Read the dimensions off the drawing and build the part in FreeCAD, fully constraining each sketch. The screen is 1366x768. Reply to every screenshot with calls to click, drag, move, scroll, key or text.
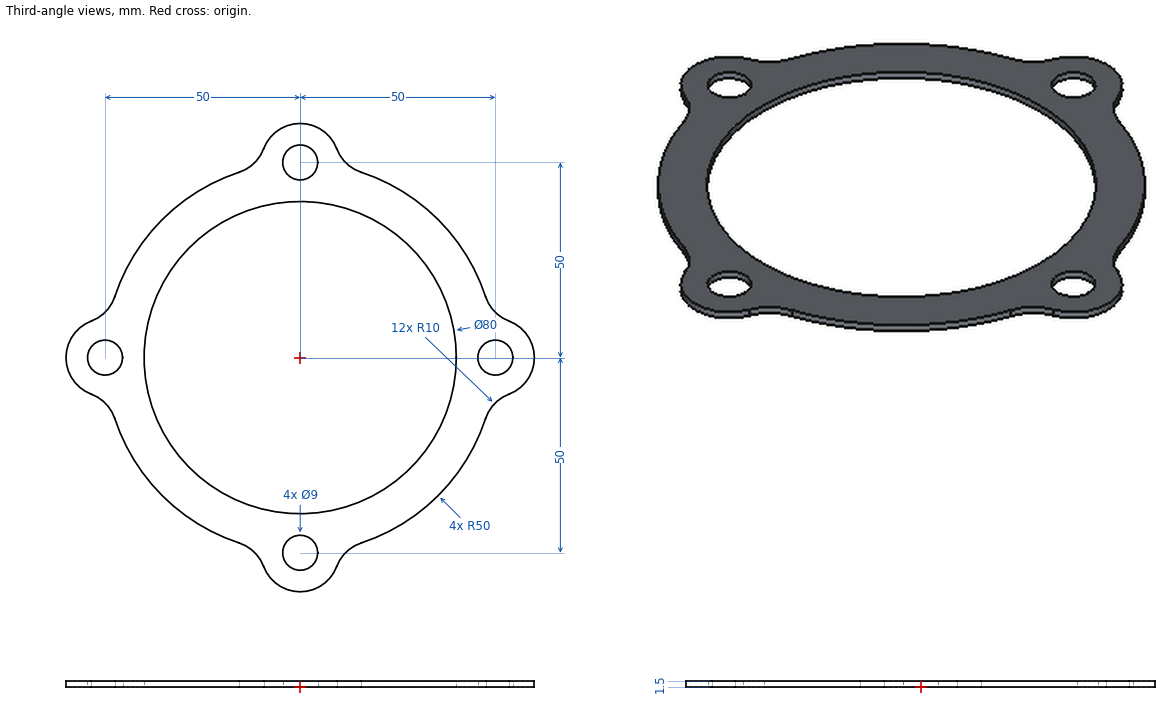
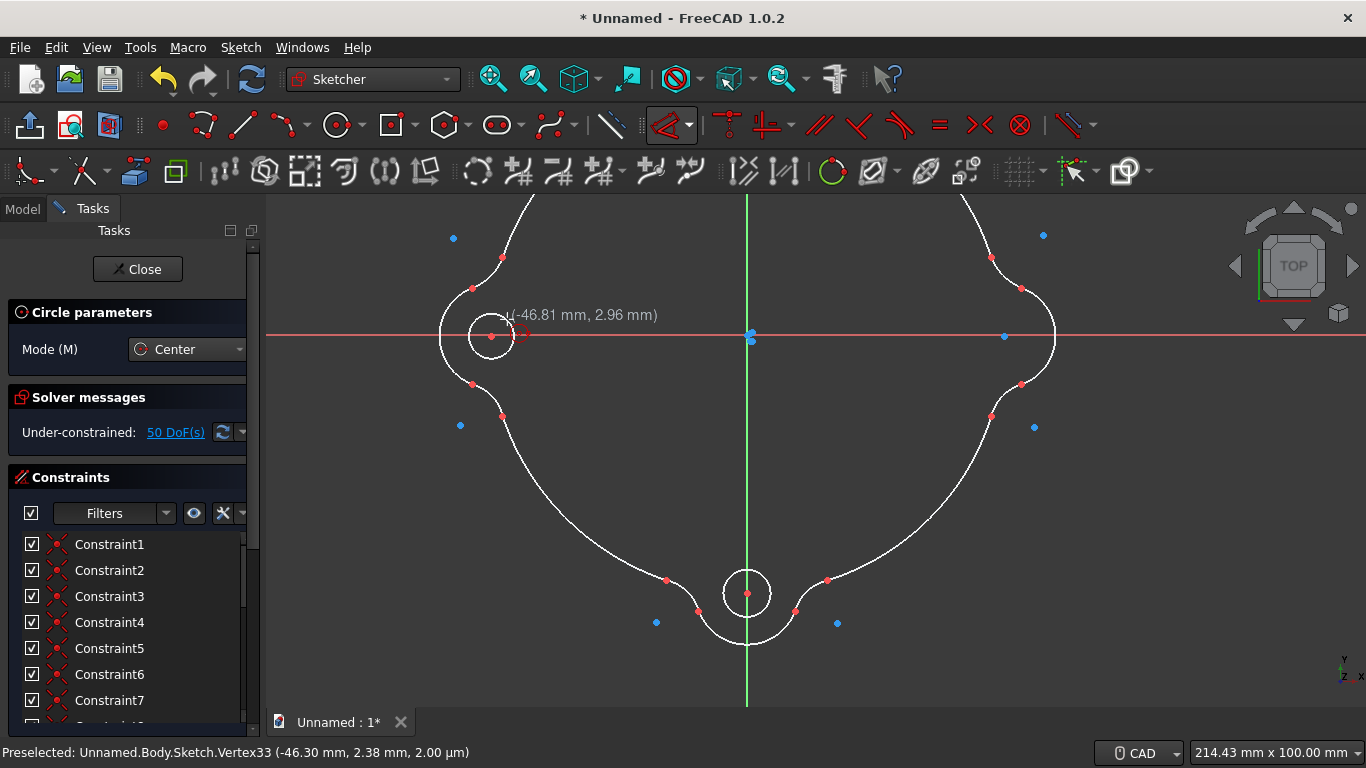
click(747, 335)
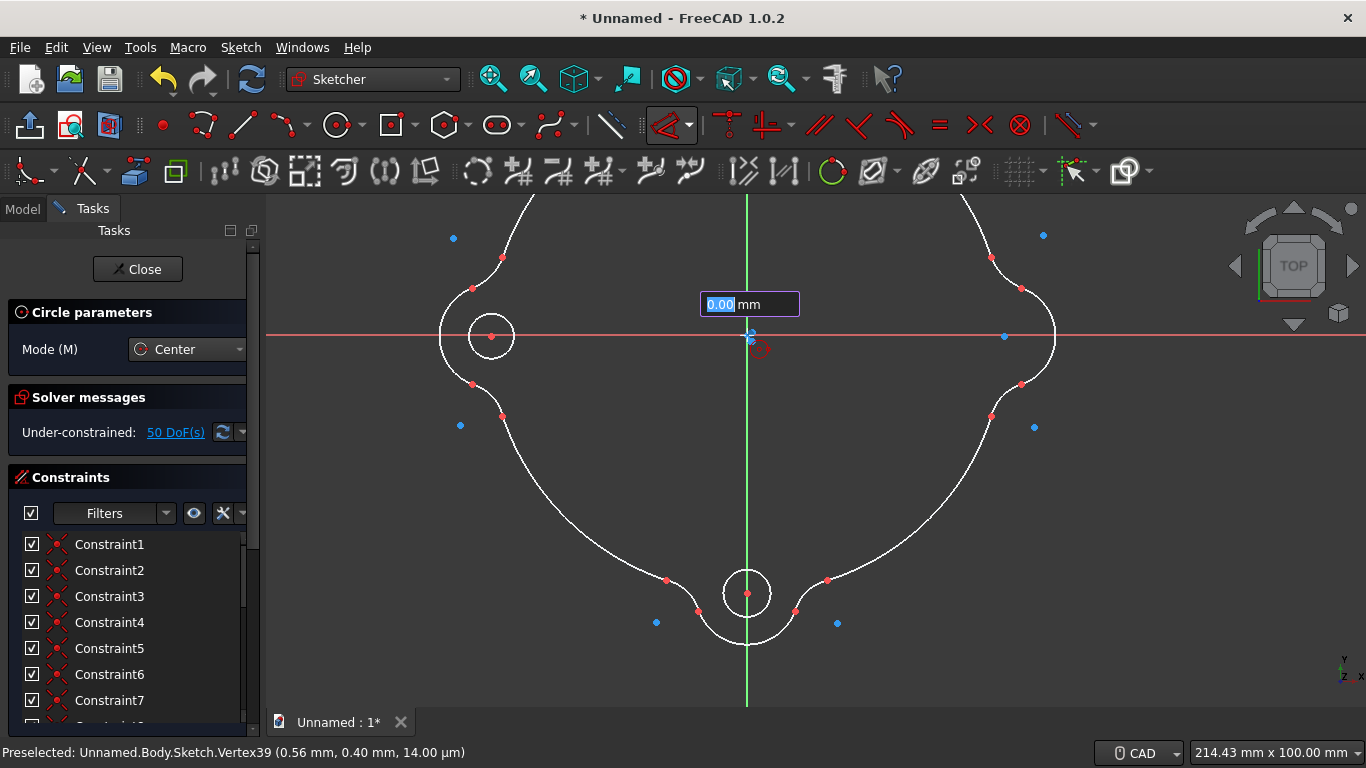
scroll(748, 591, down, 3)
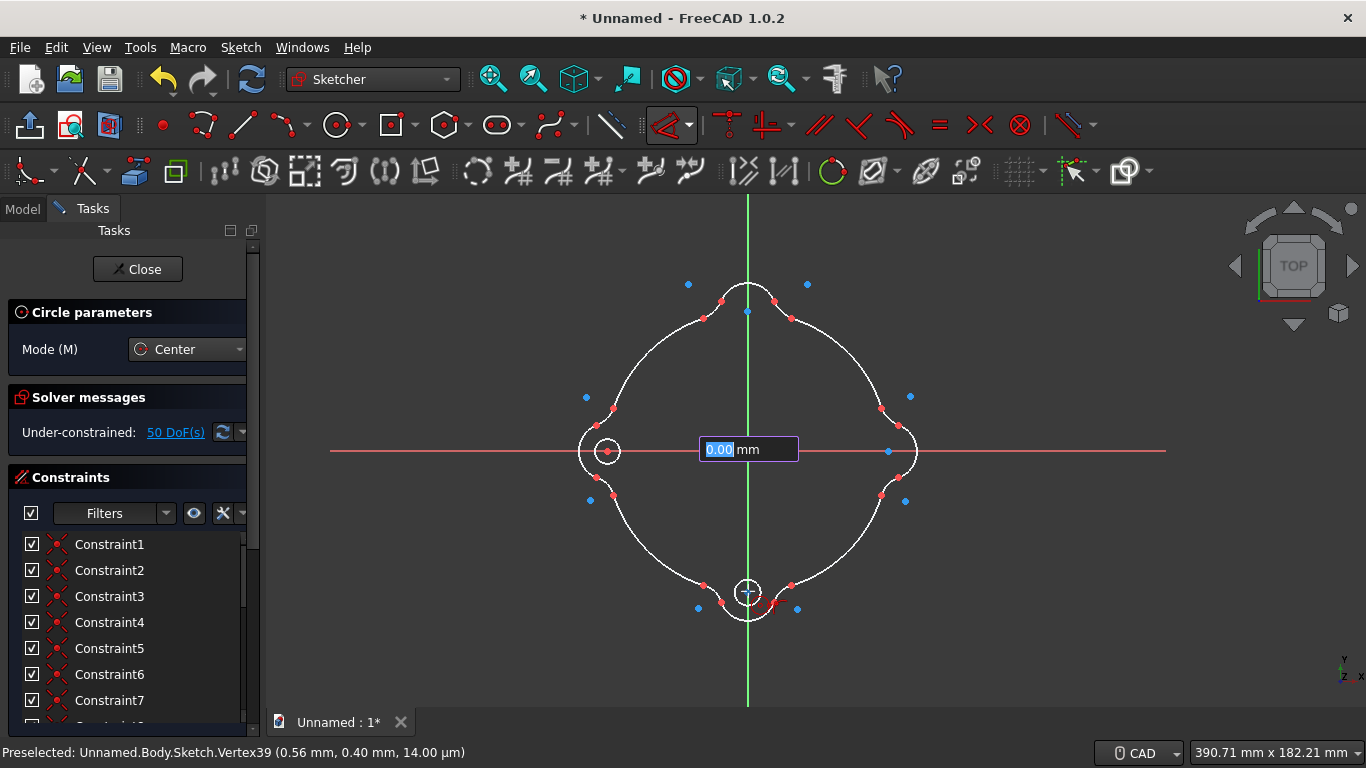
click(827, 371)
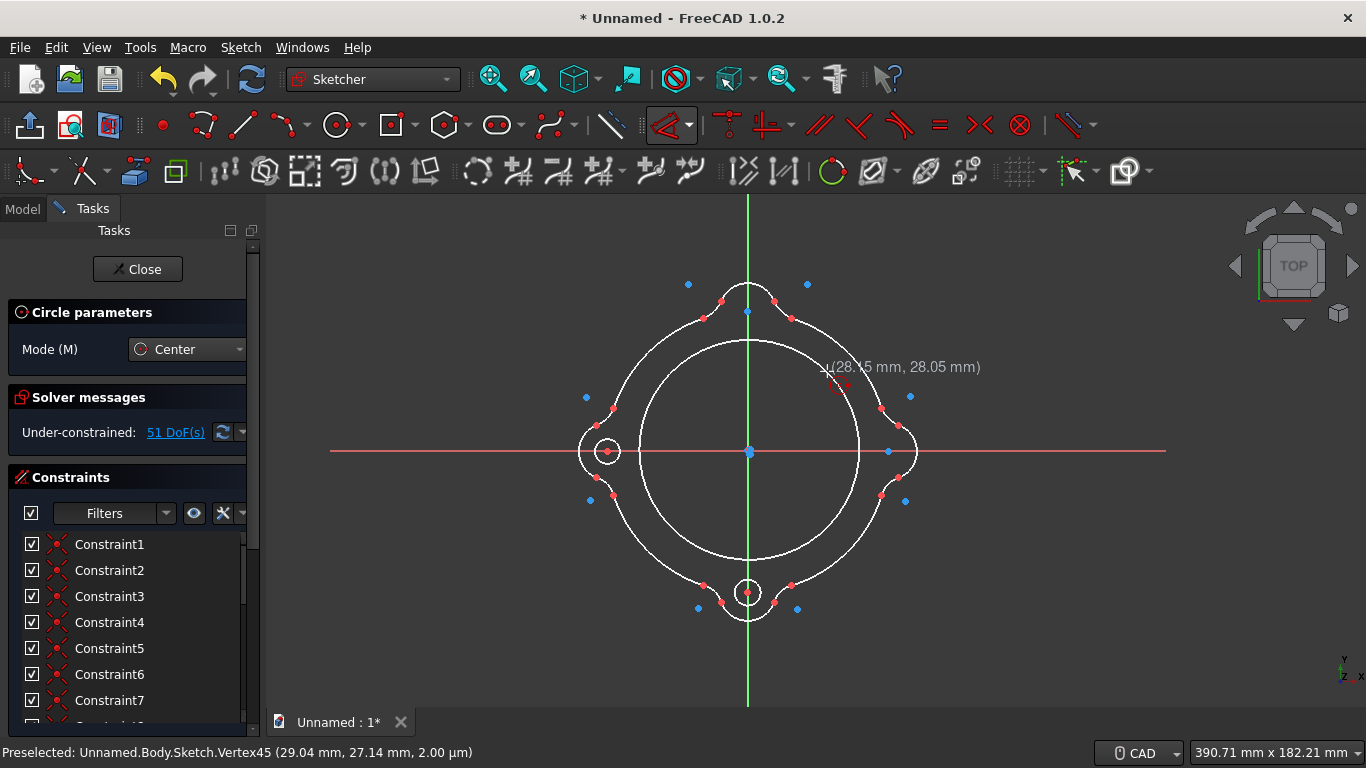
scroll(889, 451, up, 3)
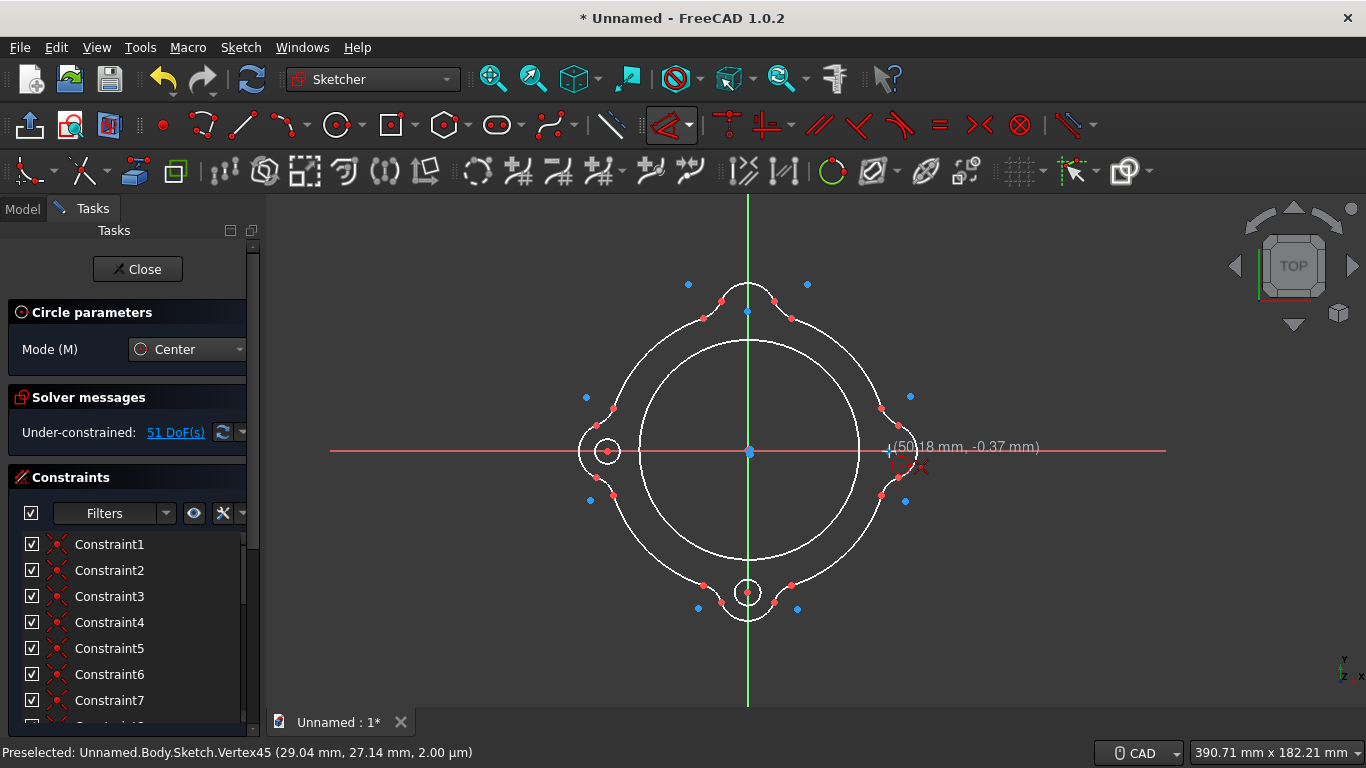
click(888, 451)
click(904, 434)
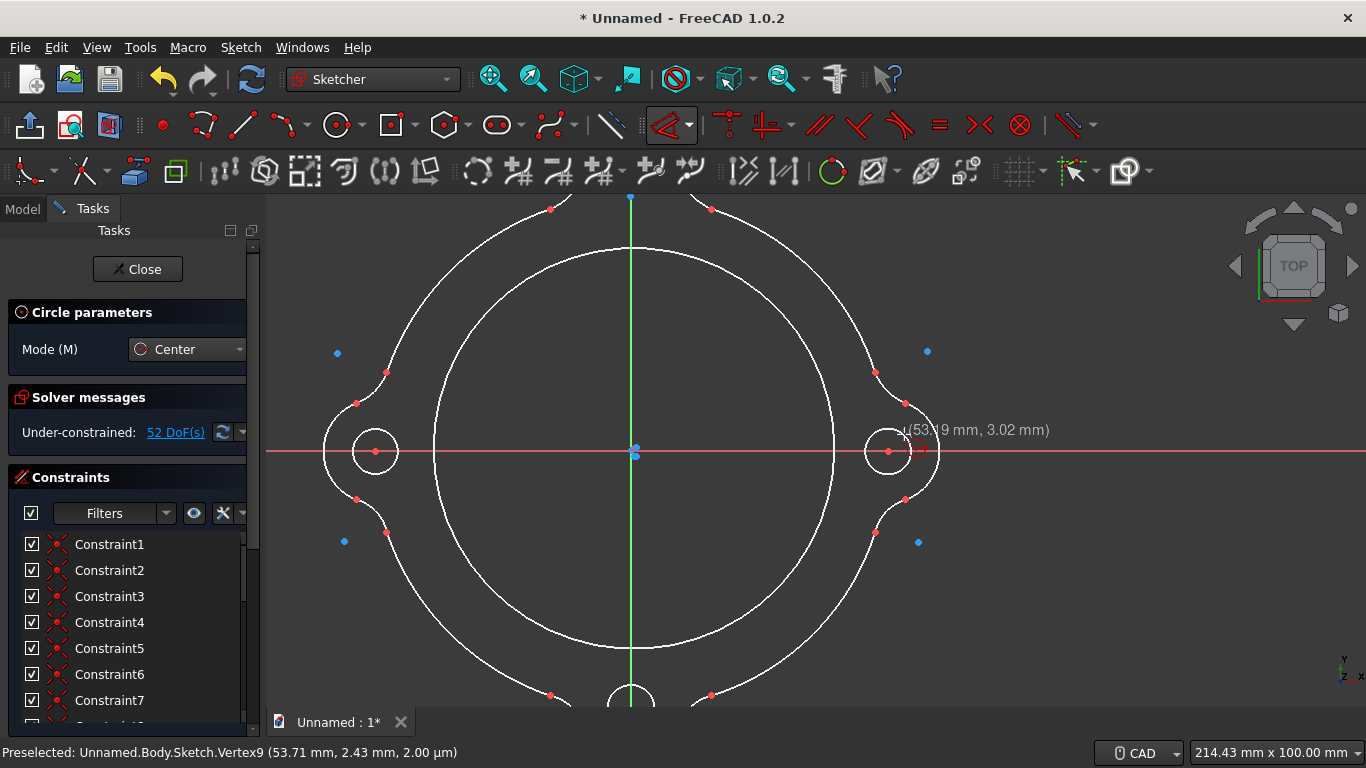
scroll(889, 450, down, 3)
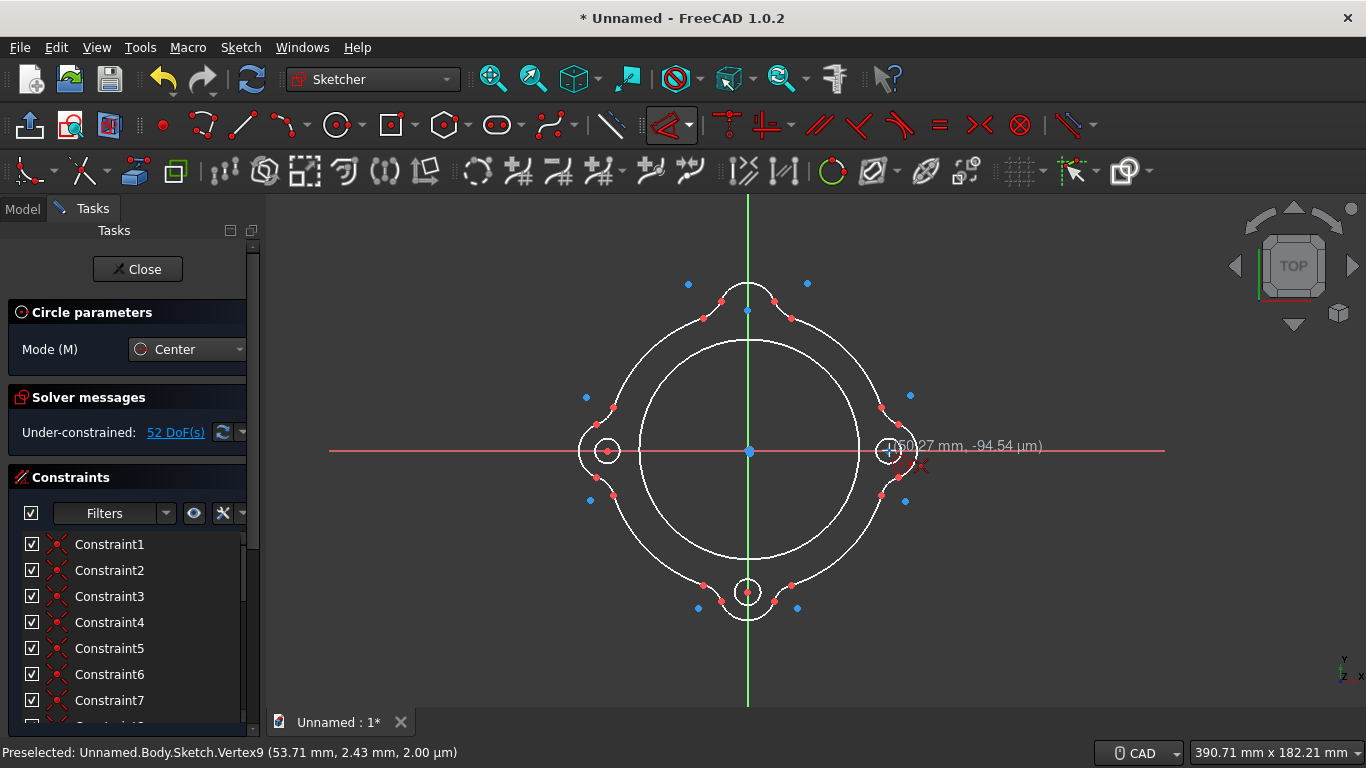
scroll(748, 310, up, 3)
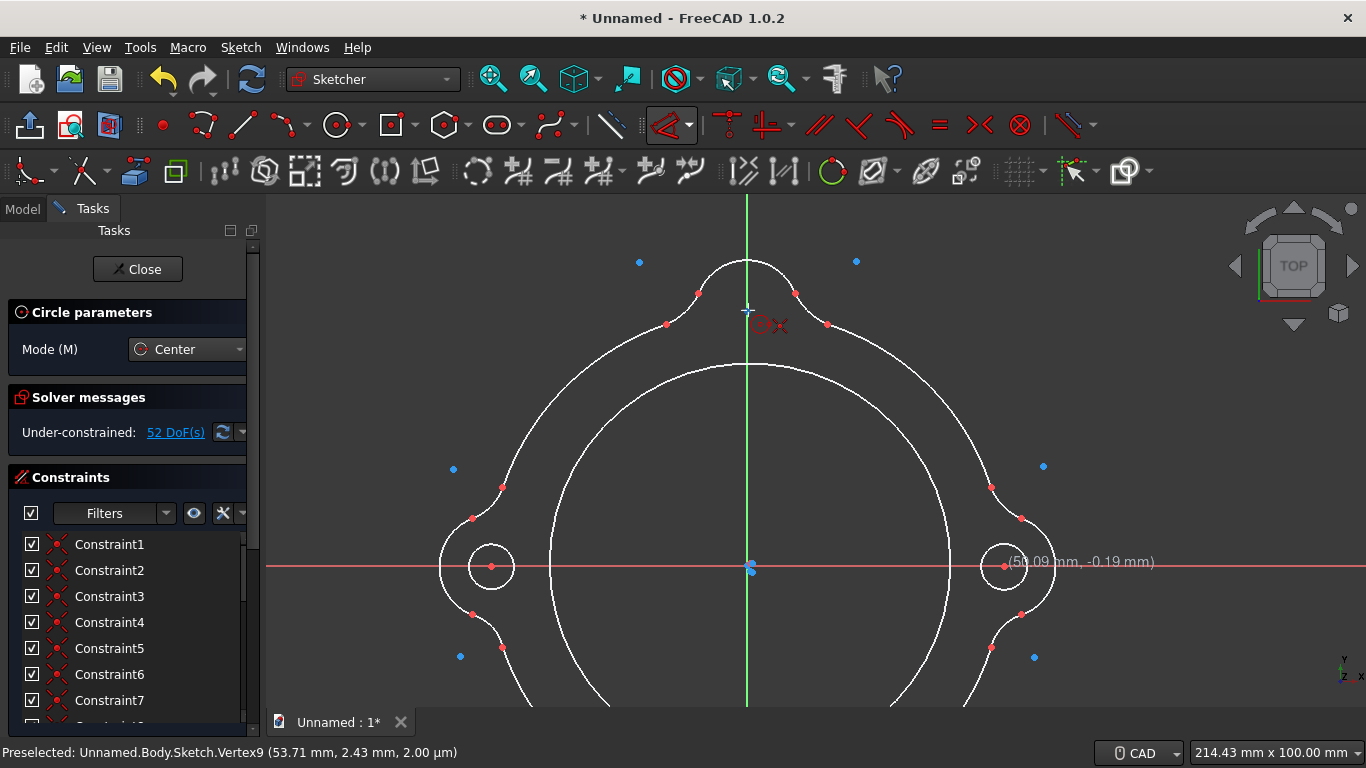
click(747, 309)
click(763, 293)
key(Escape)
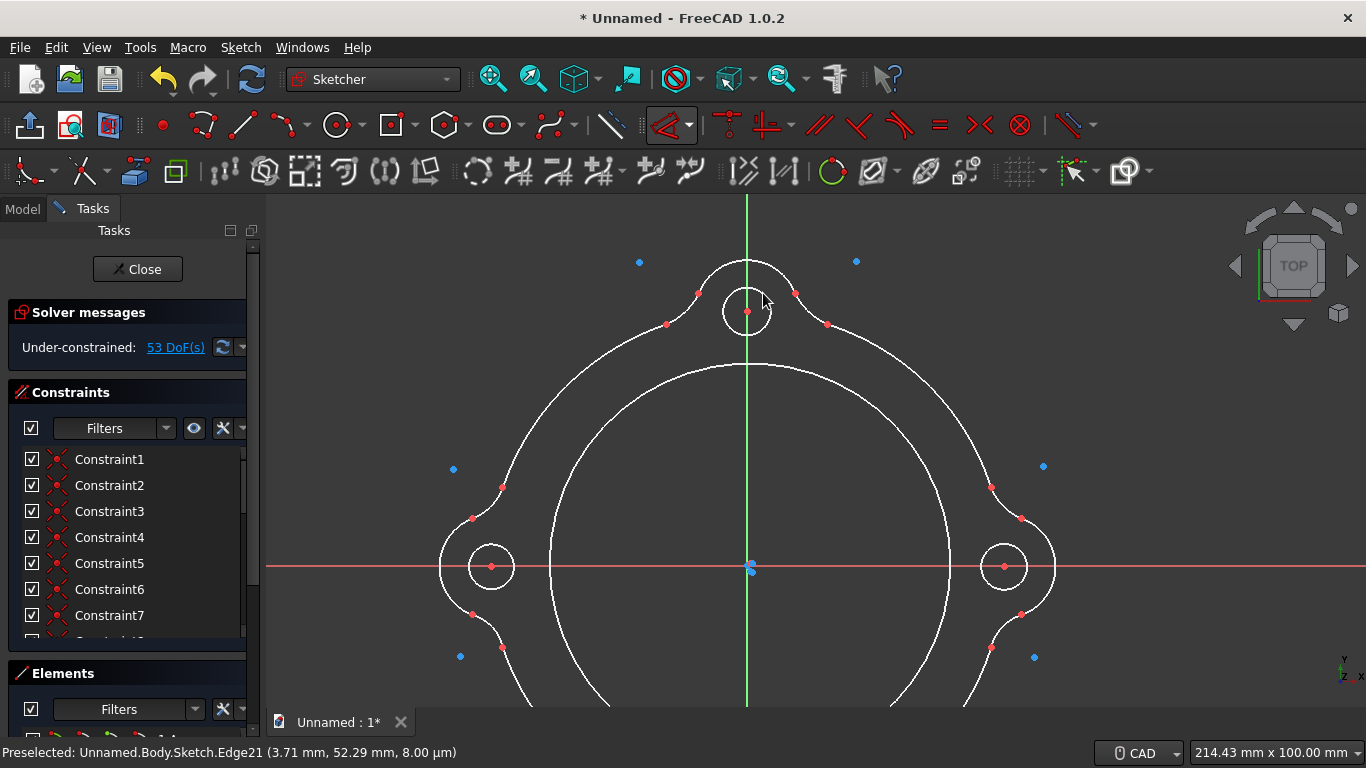
scroll(748, 310, down, 3)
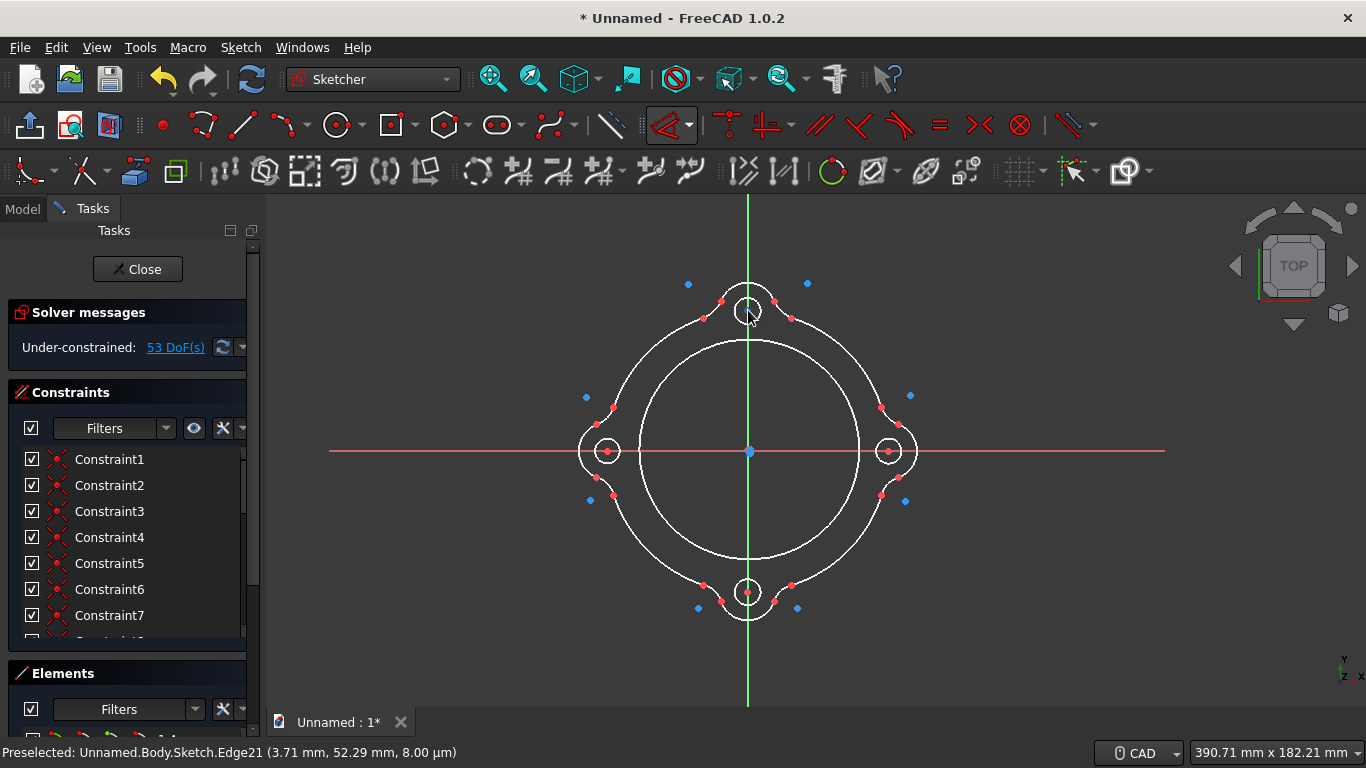
click(827, 568)